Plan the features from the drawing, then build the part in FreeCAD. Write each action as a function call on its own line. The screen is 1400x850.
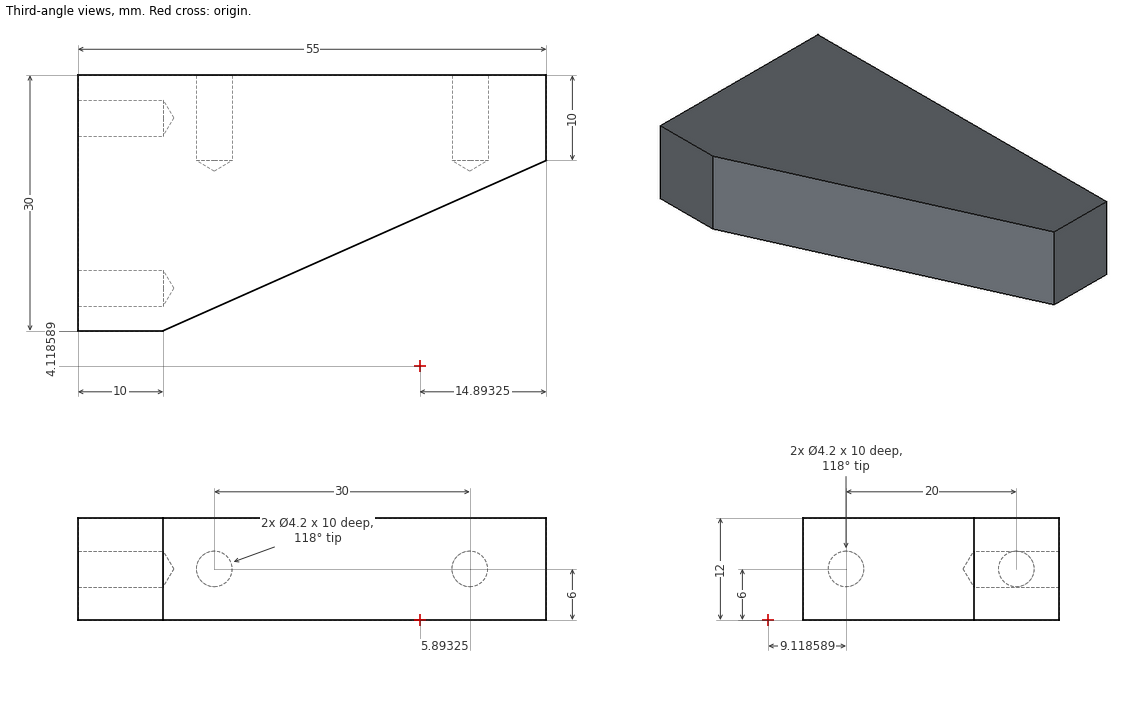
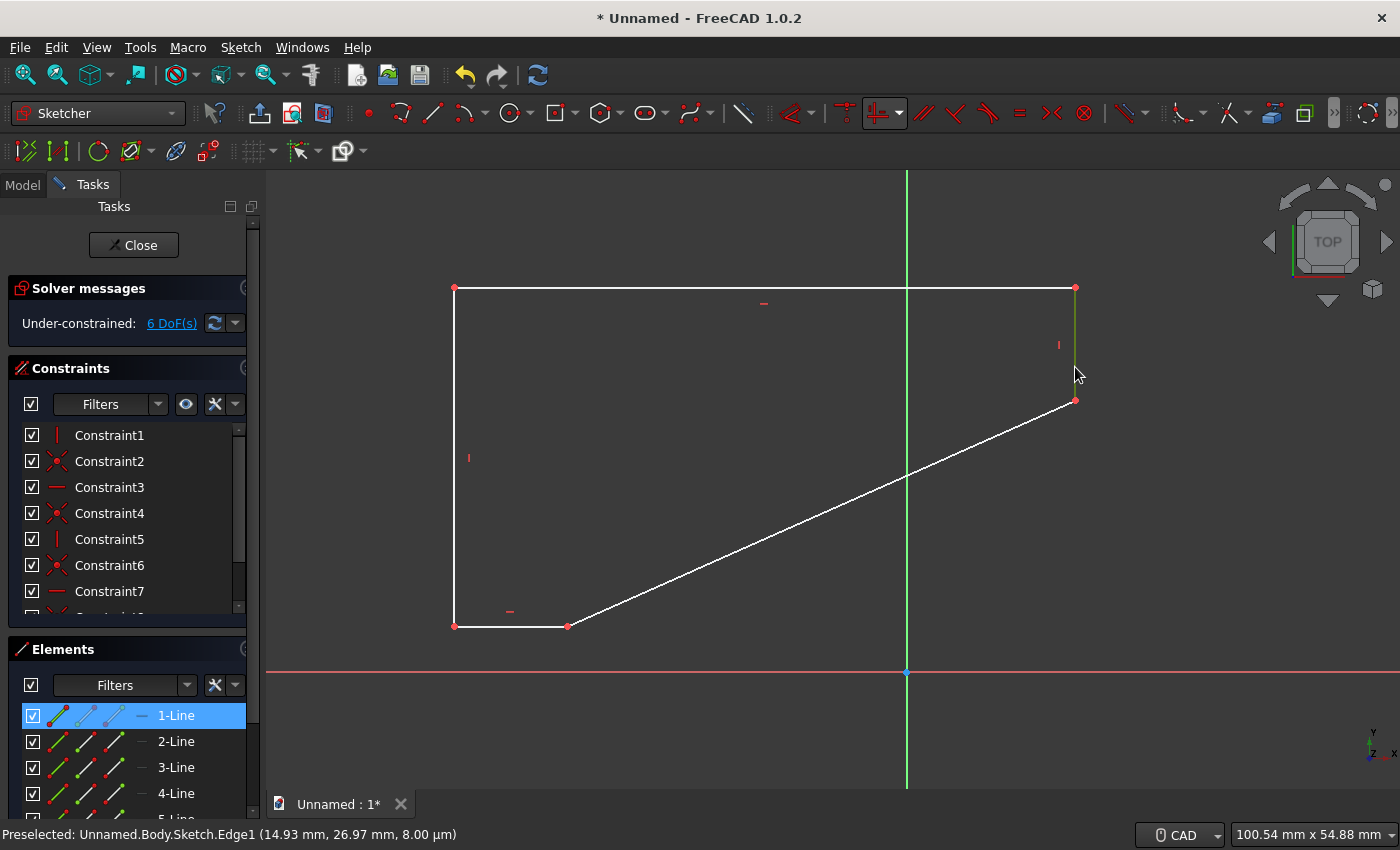
click(814, 114)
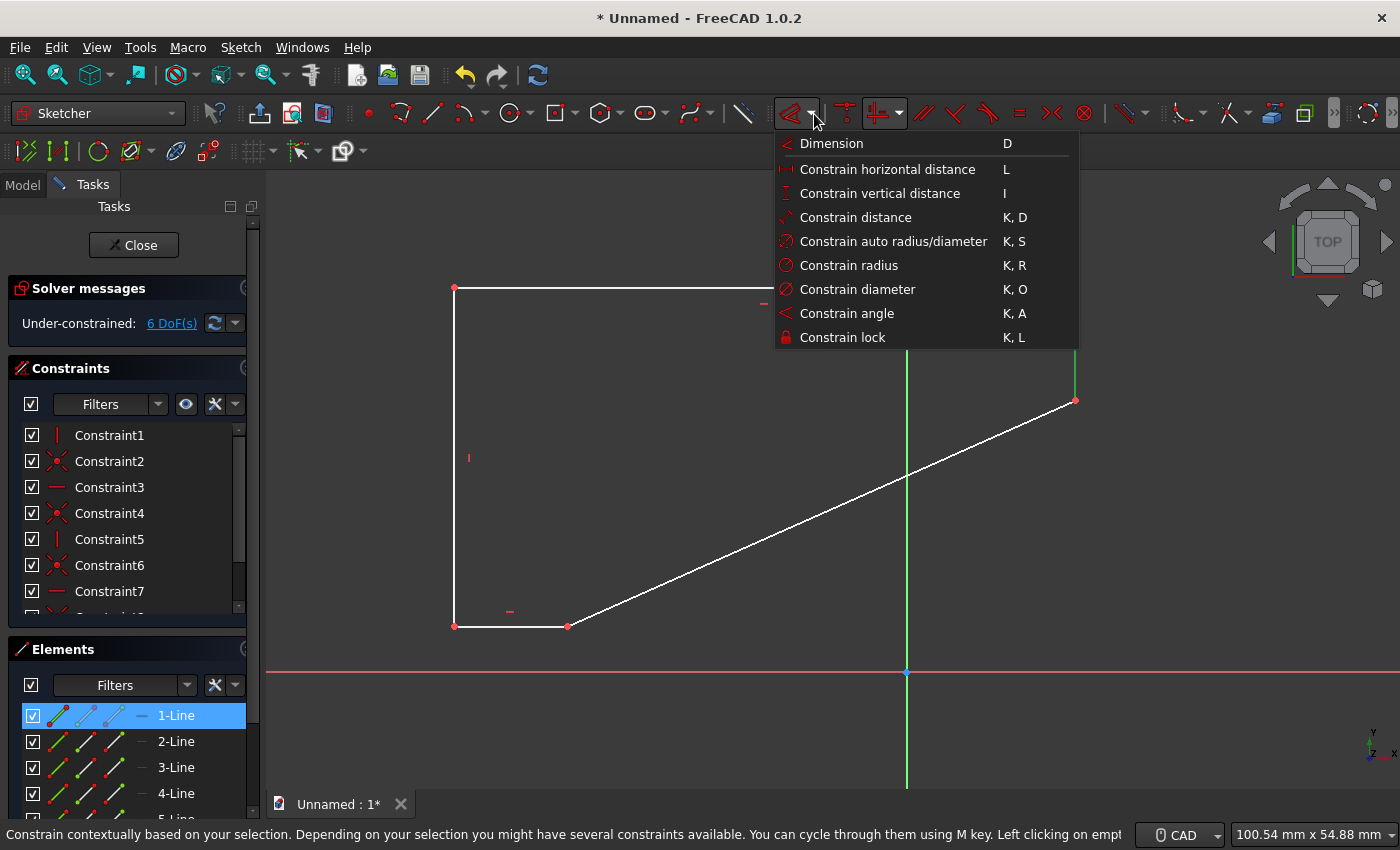
click(927, 193)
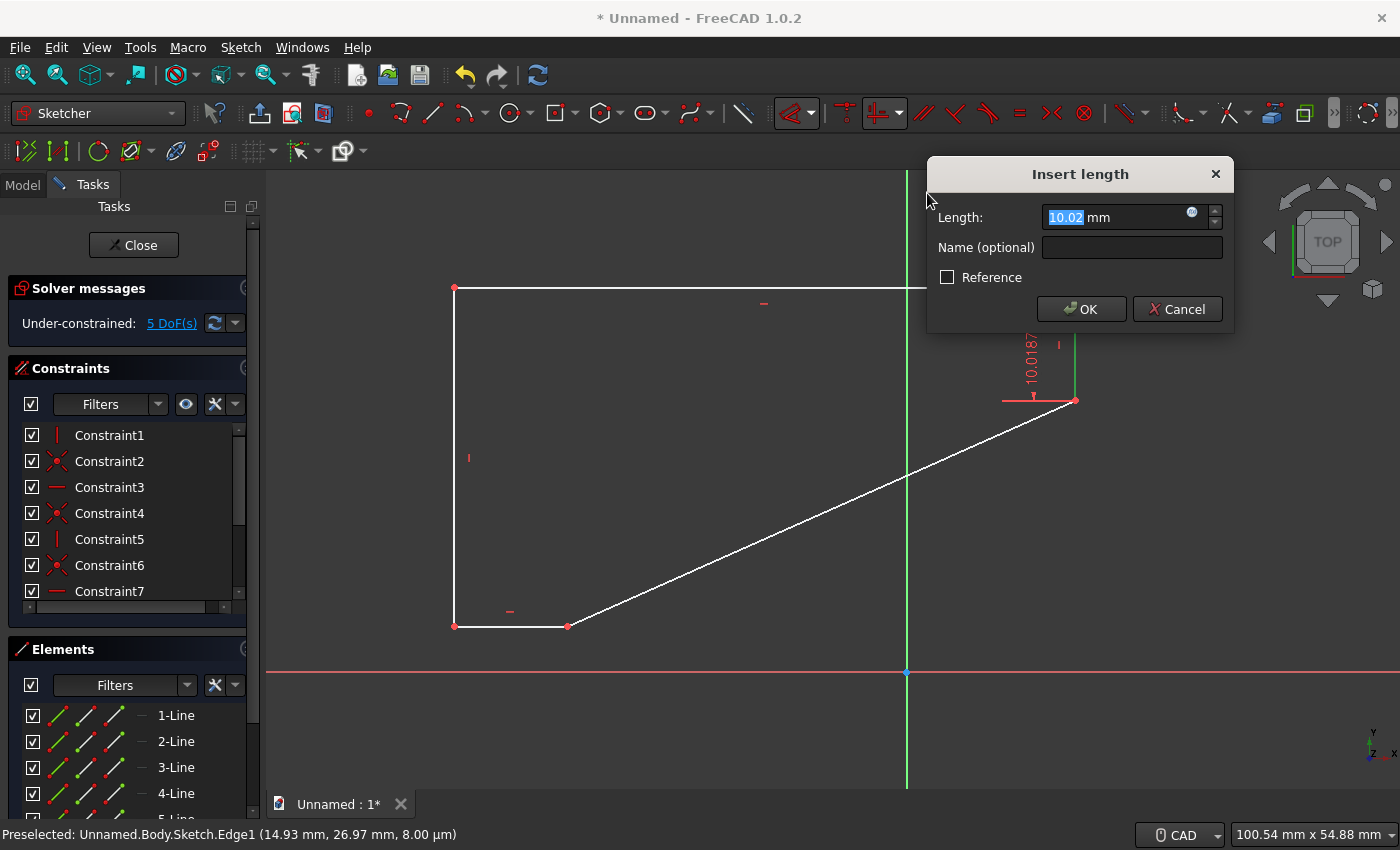
text(10)
key(Return)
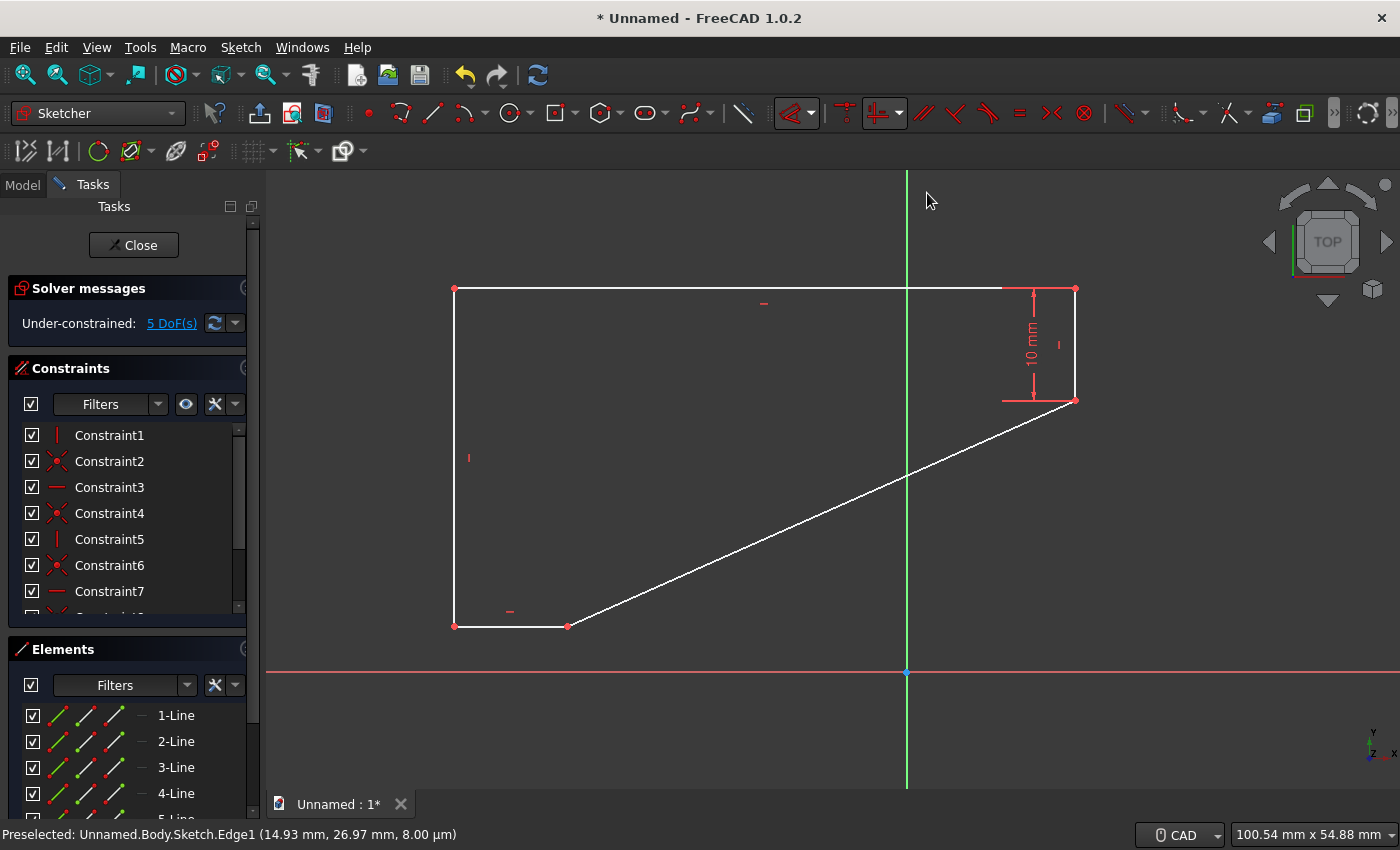
click(889, 288)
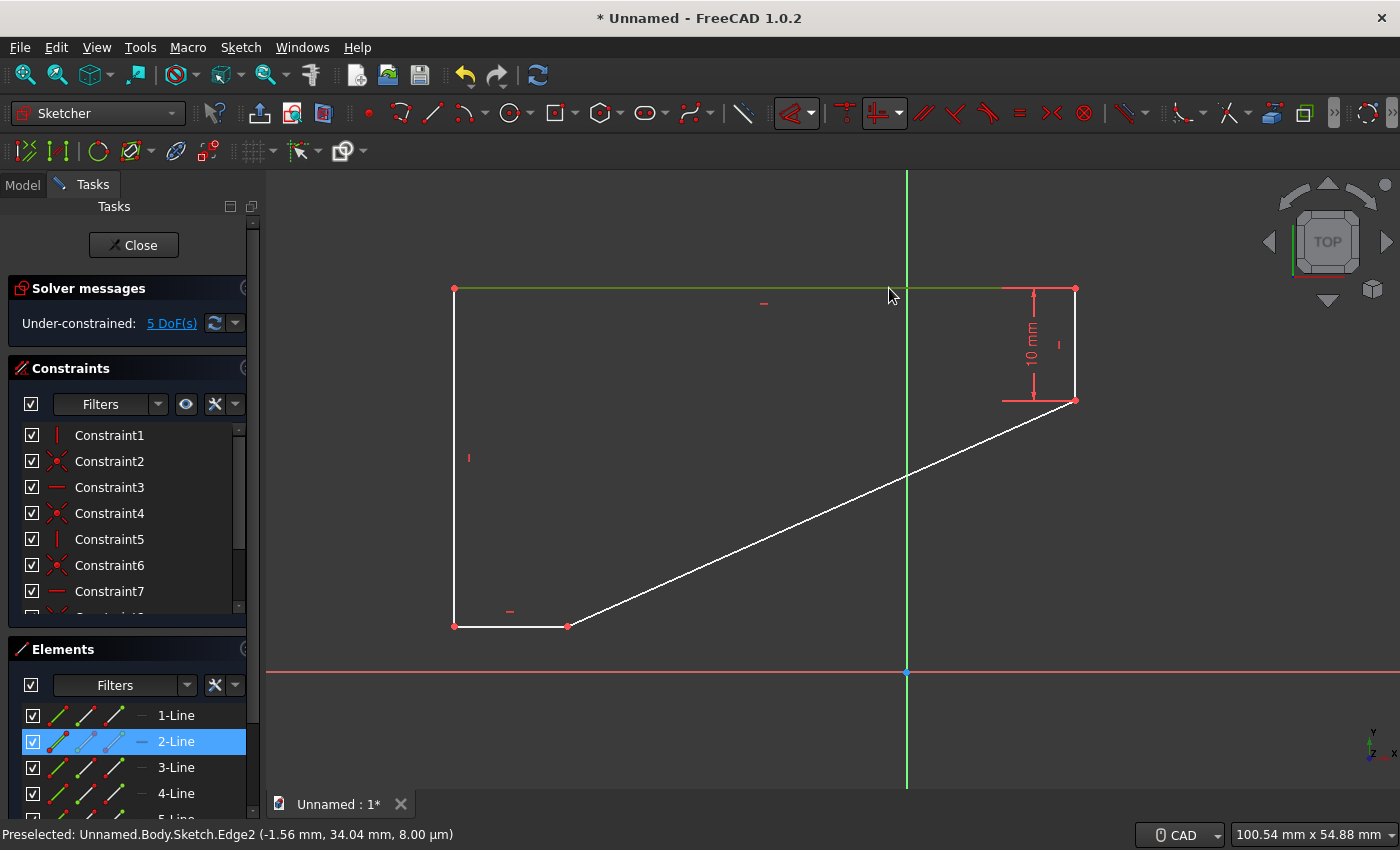
key(l)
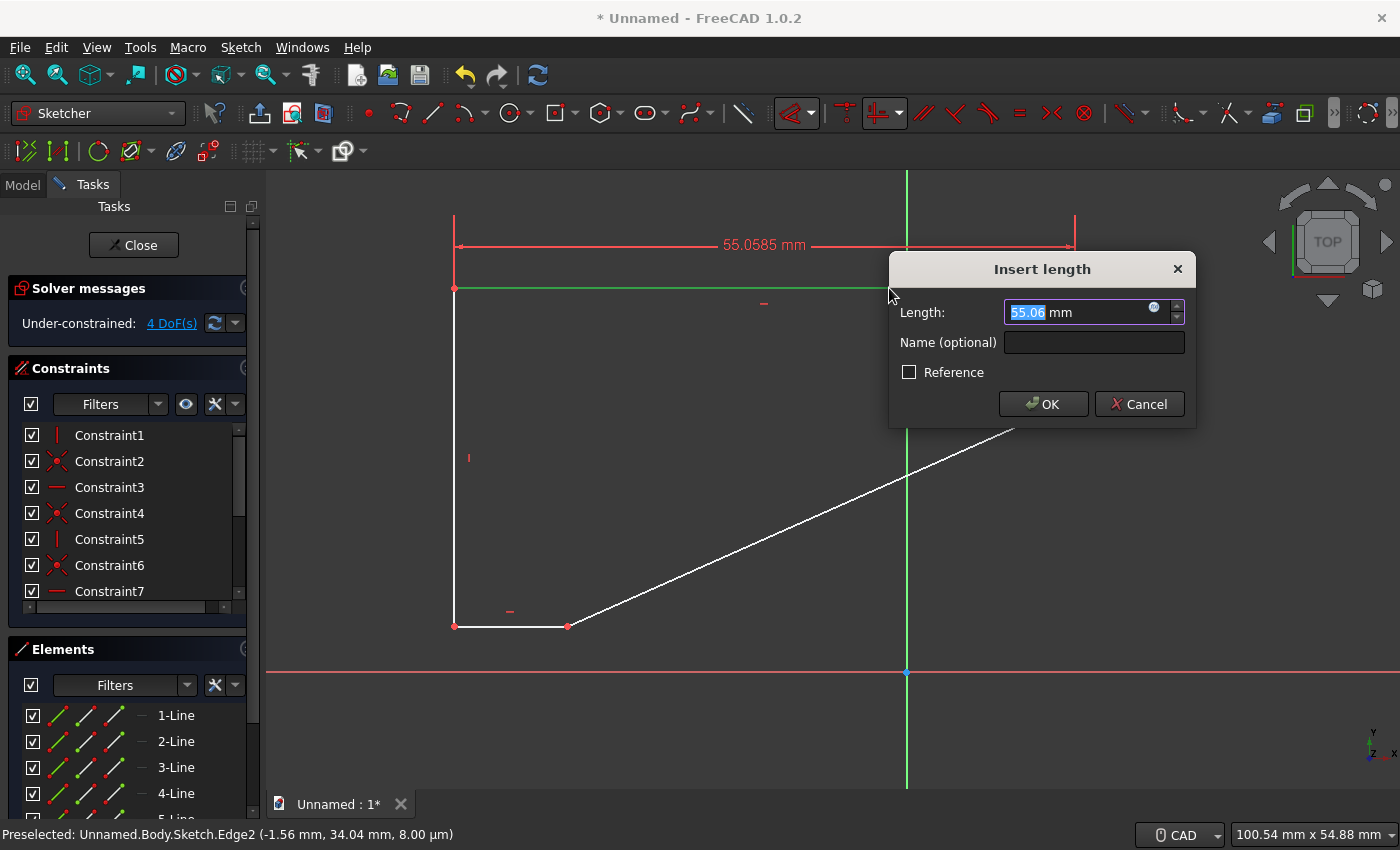
text(55)
key(Return)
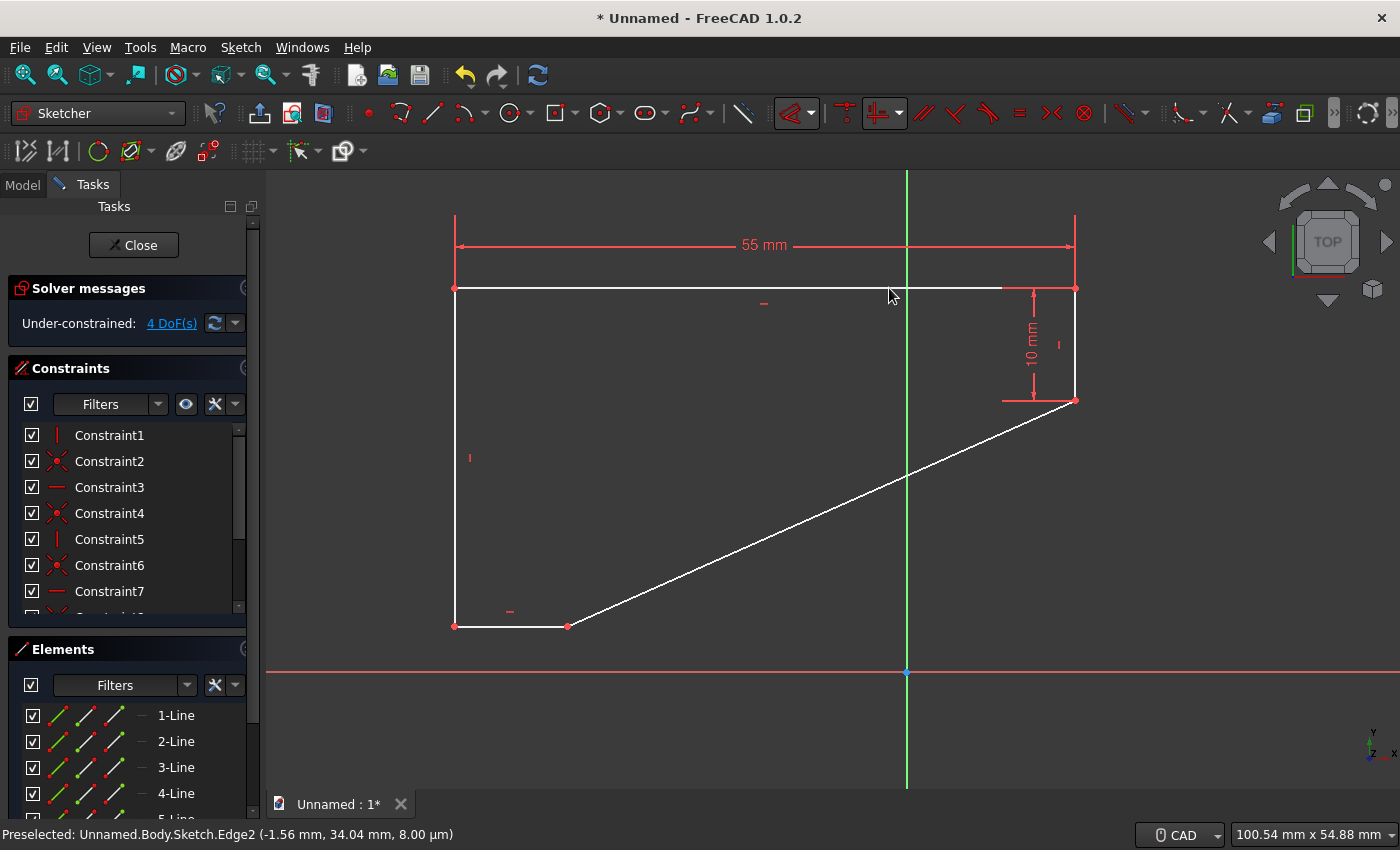
click(455, 390)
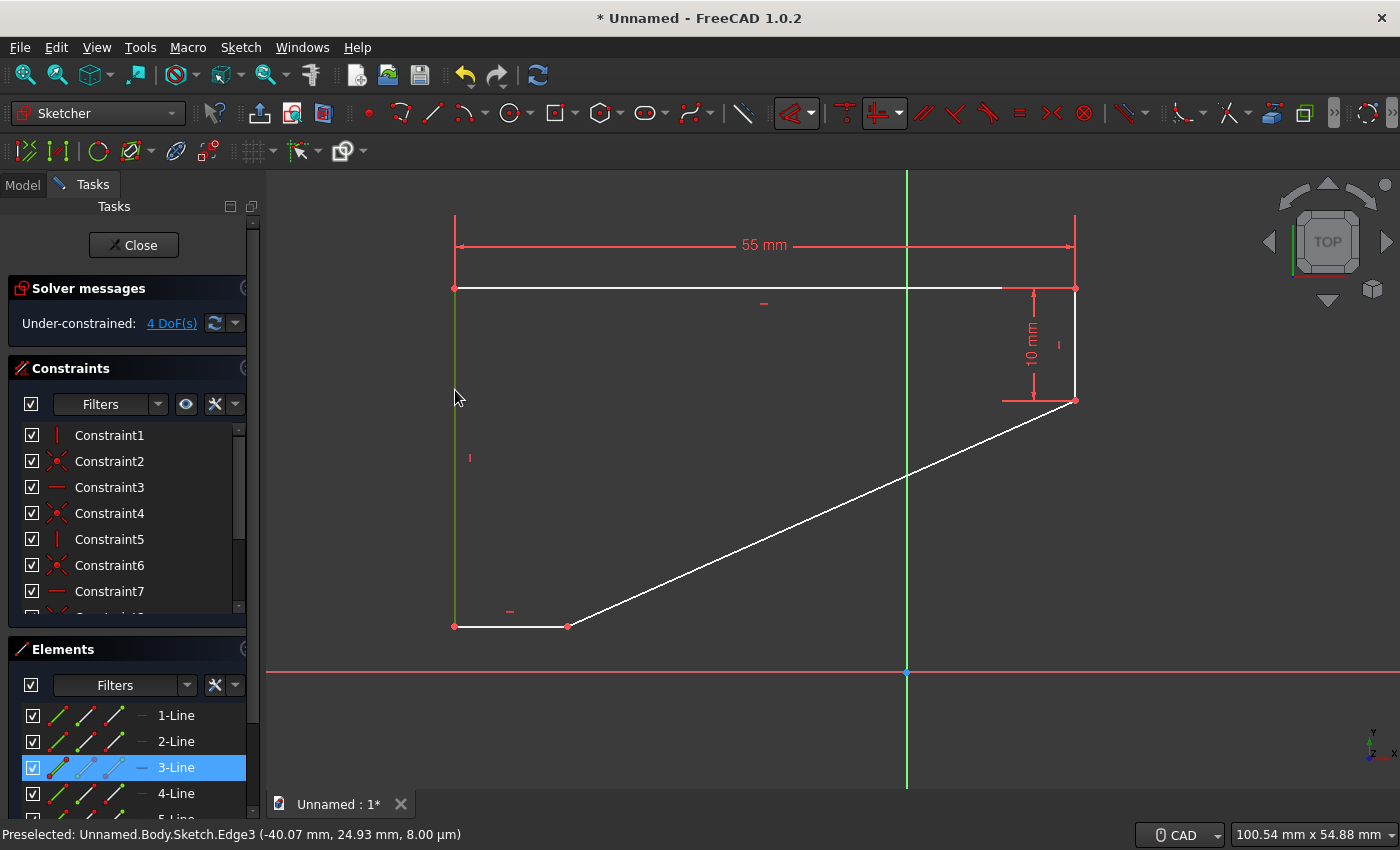
key(i)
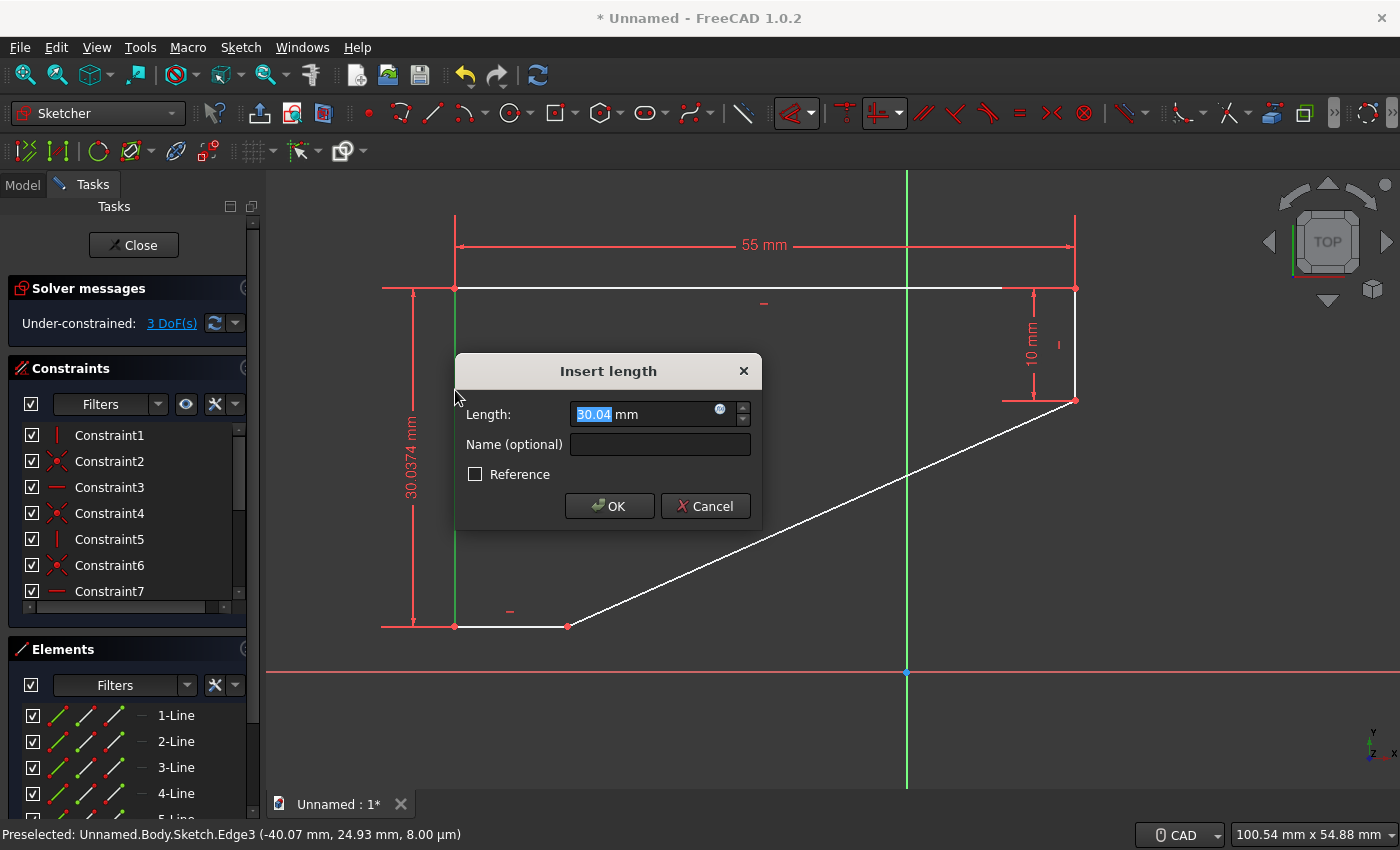
text(30)
key(Return)